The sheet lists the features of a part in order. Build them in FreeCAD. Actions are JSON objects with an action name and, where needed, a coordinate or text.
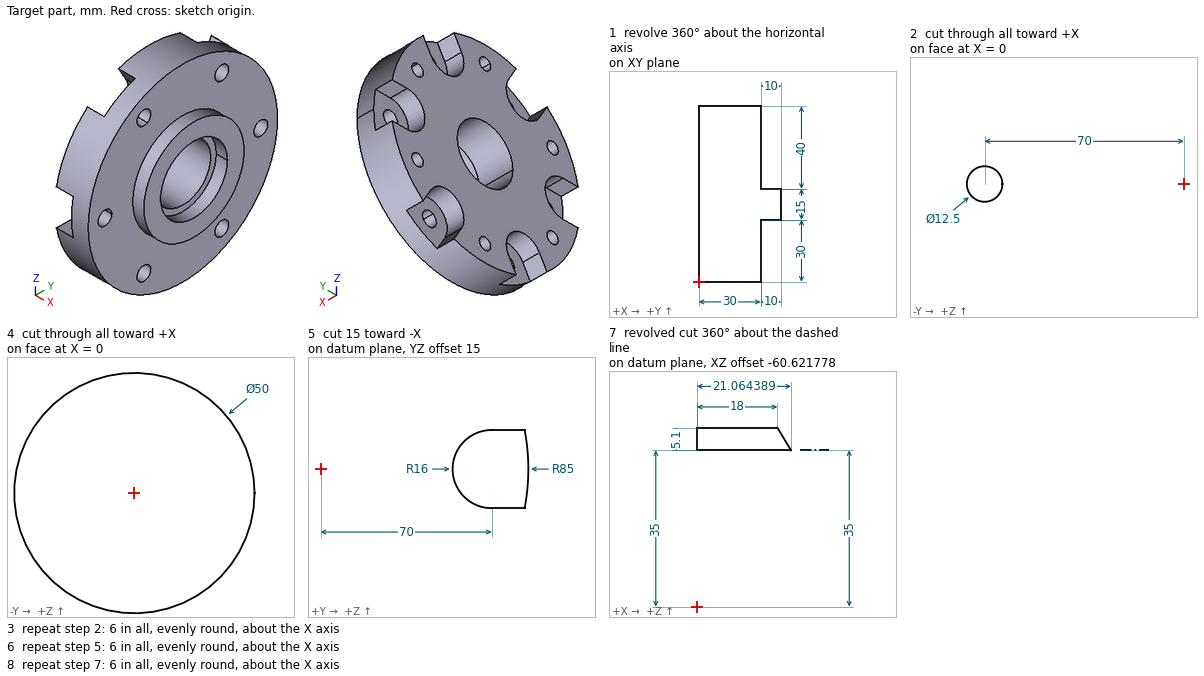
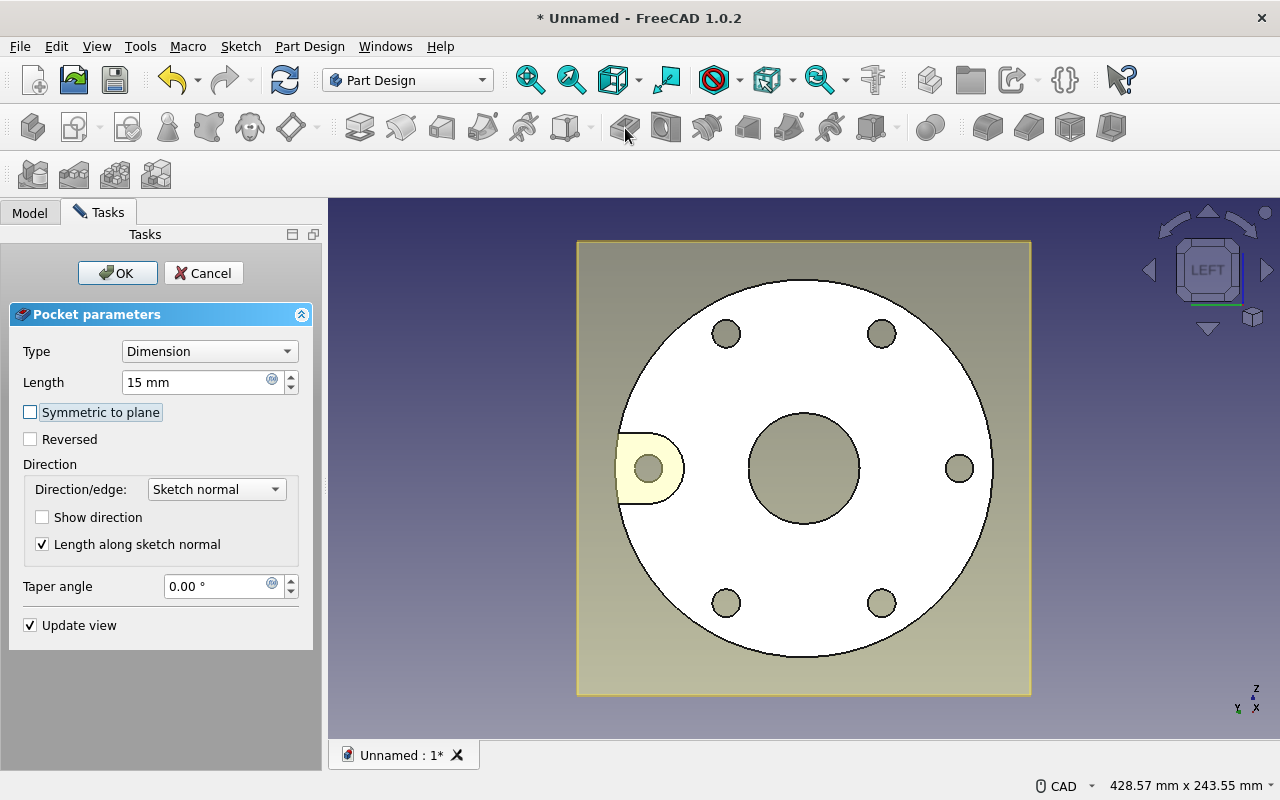
{"action": "left_click", "coordinate": [118, 273]}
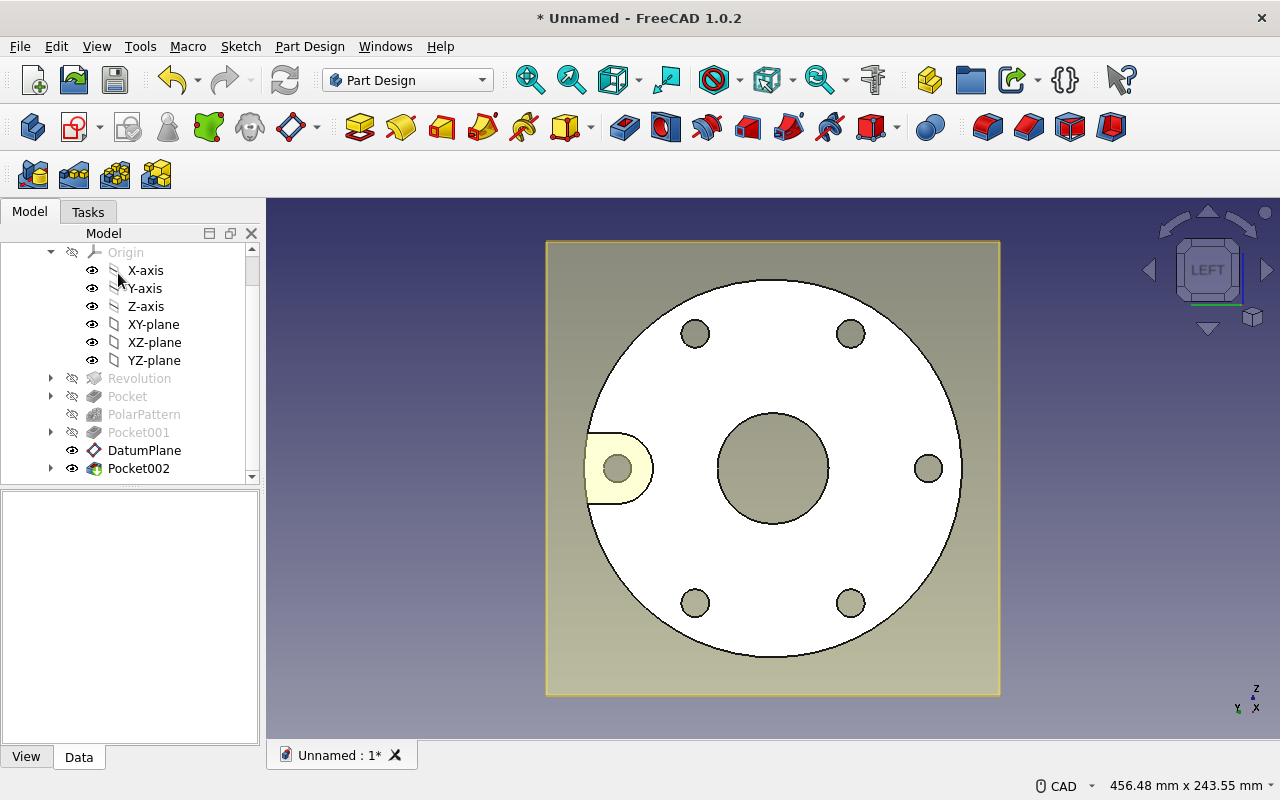
{"action": "left_click", "coordinate": [117, 450]}
{"action": "key", "text": "space"}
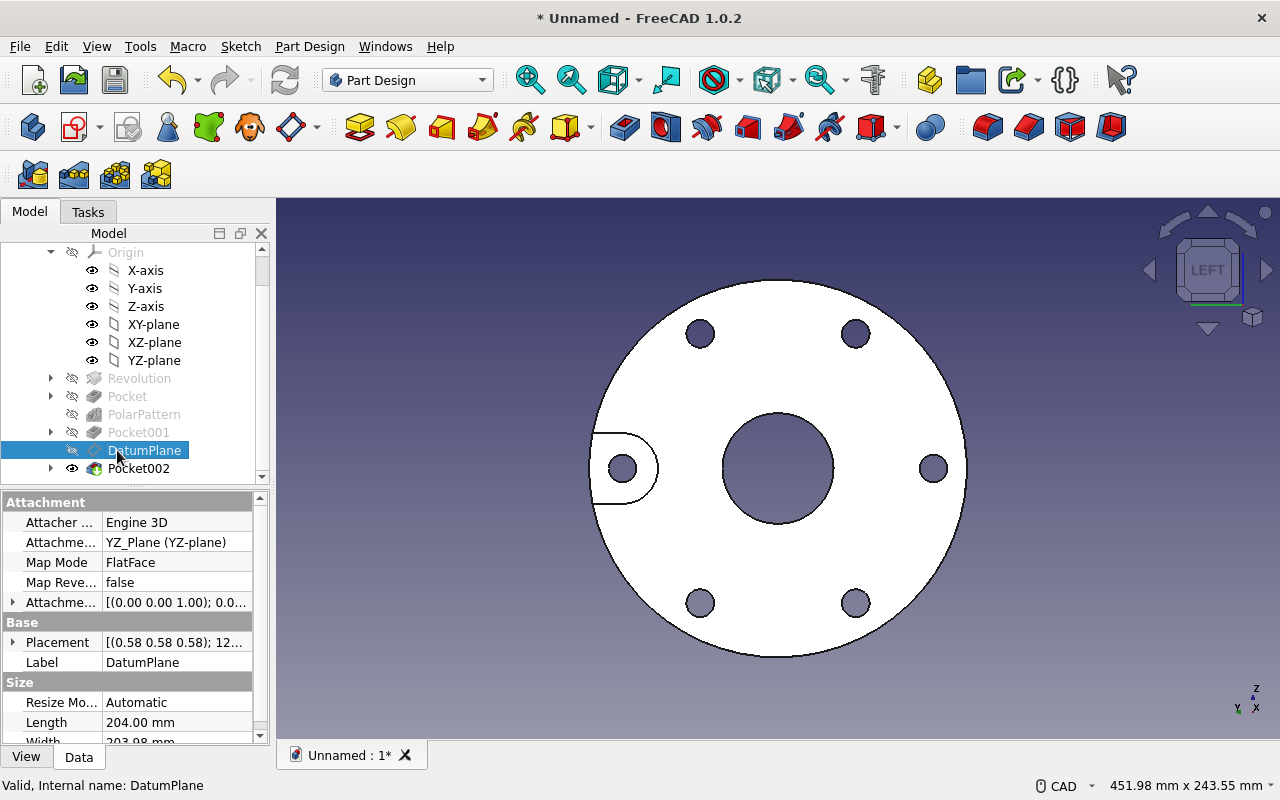
{"action": "left_click", "coordinate": [117, 468]}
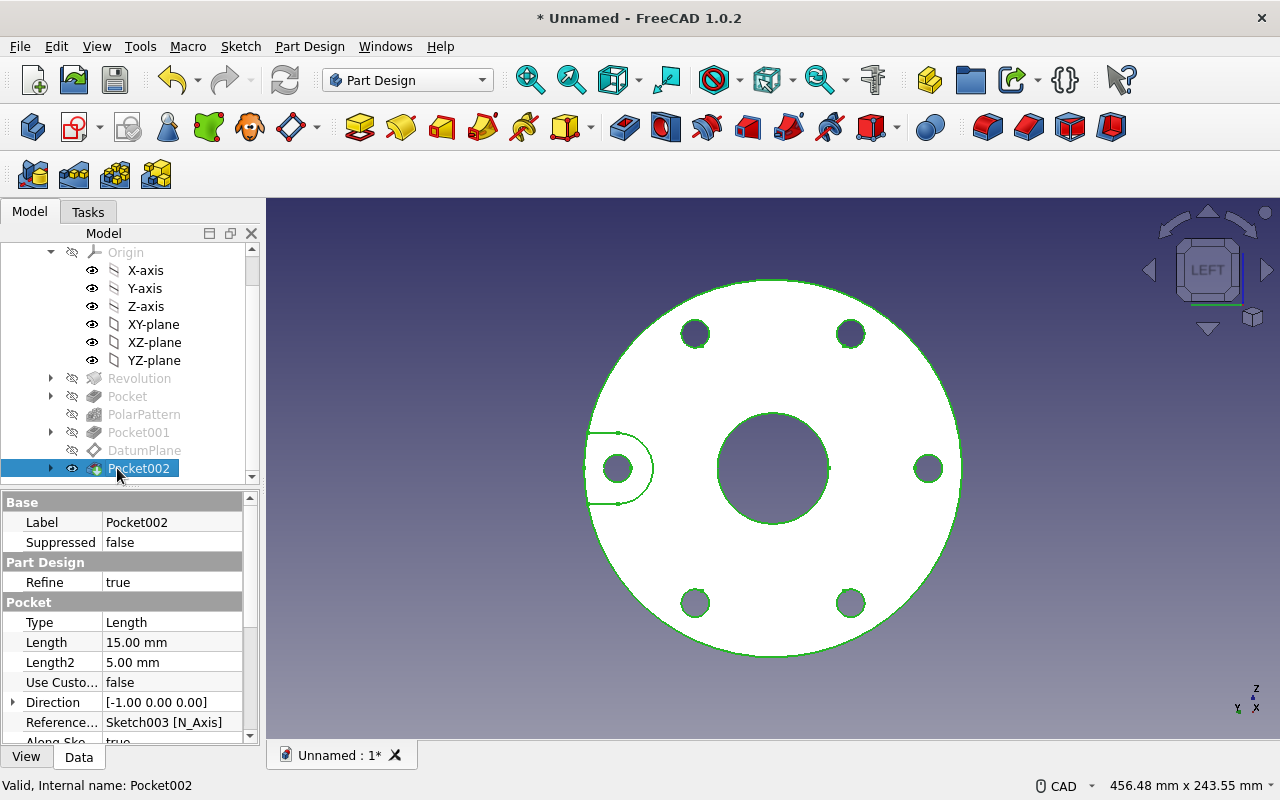
{"action": "left_click", "coordinate": [115, 174]}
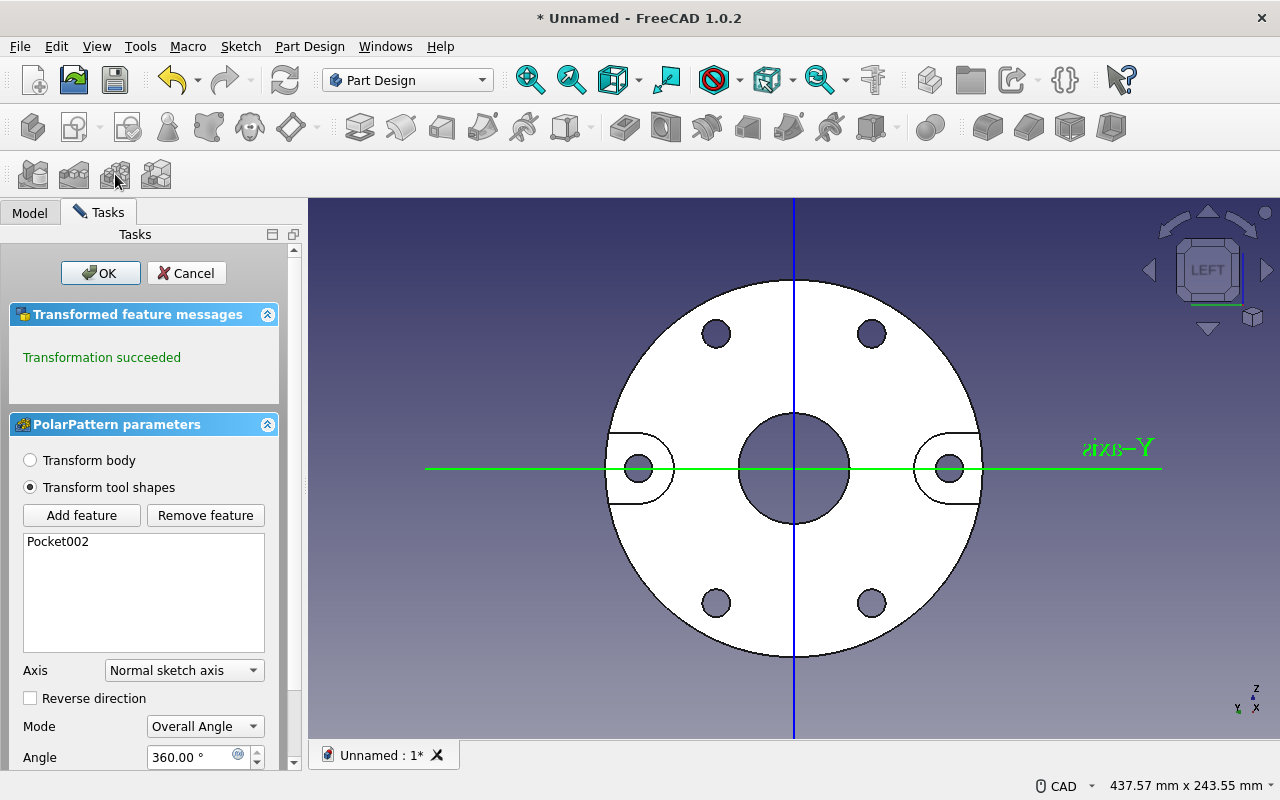
{"action": "left_click", "coordinate": [185, 670]}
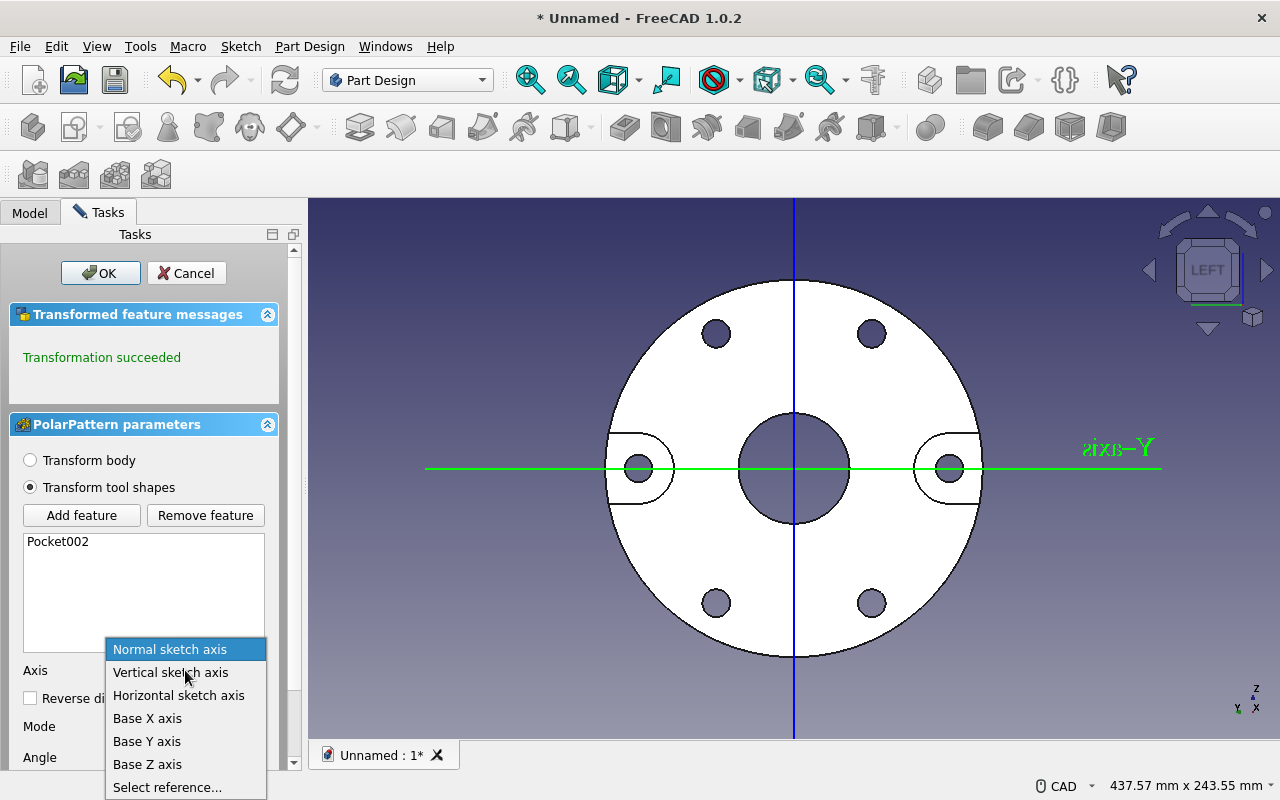
{"action": "left_click", "coordinate": [184, 718]}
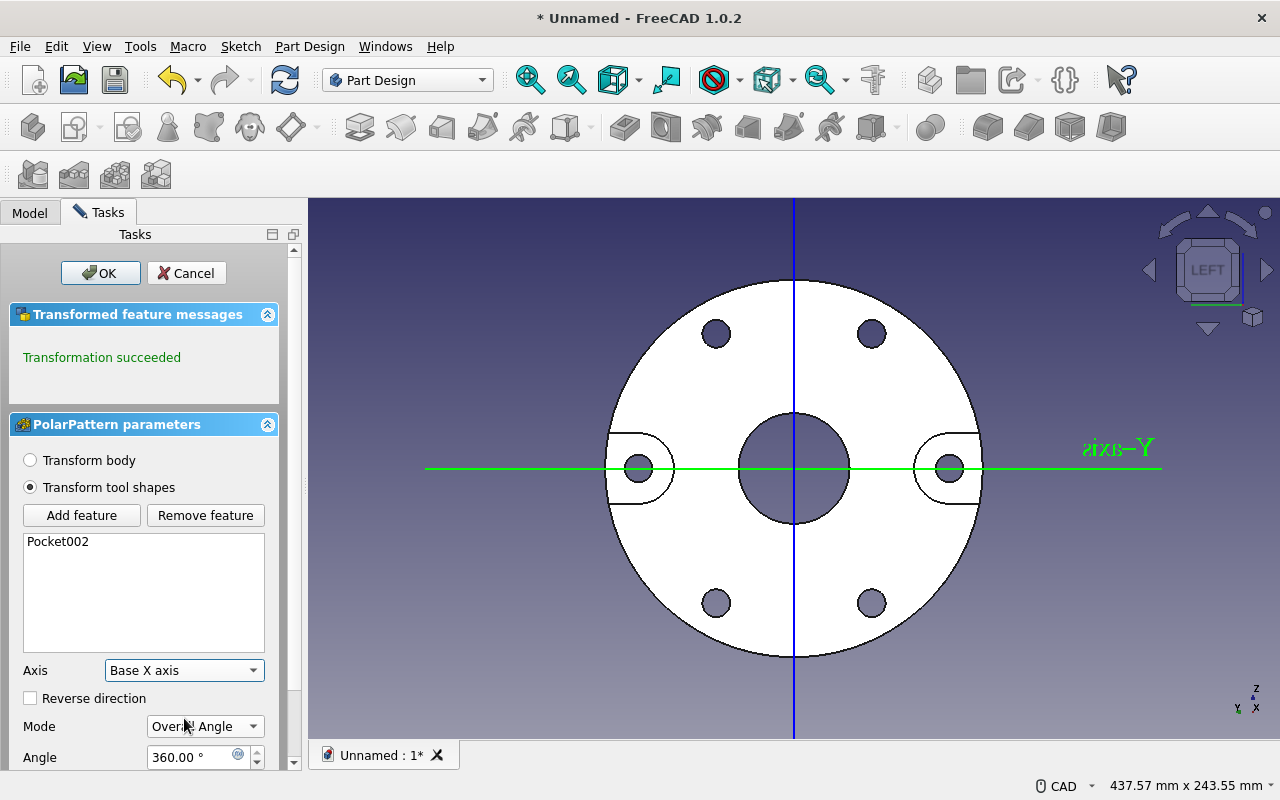
{"action": "scroll", "coordinate": [294, 507], "scroll_direction": "down", "scroll_amount": 2}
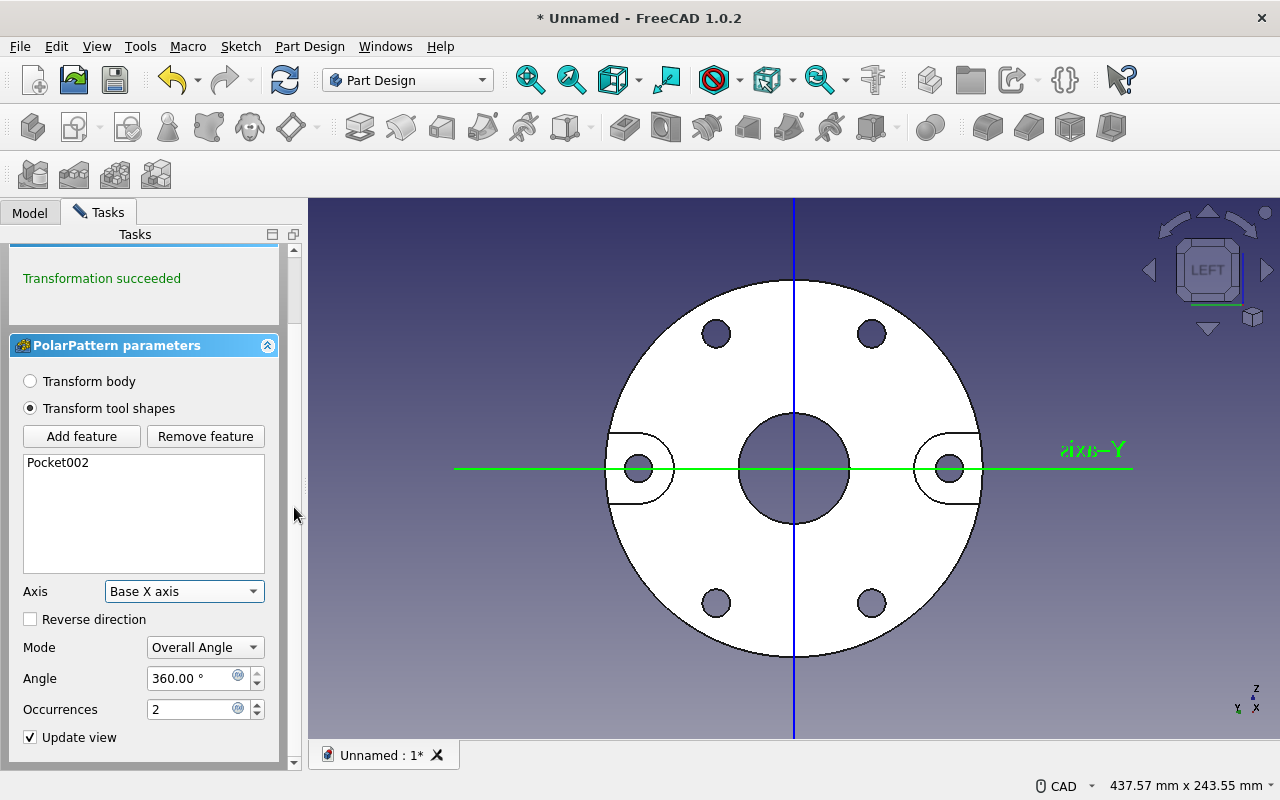
{"action": "triple_click", "coordinate": [199, 710]}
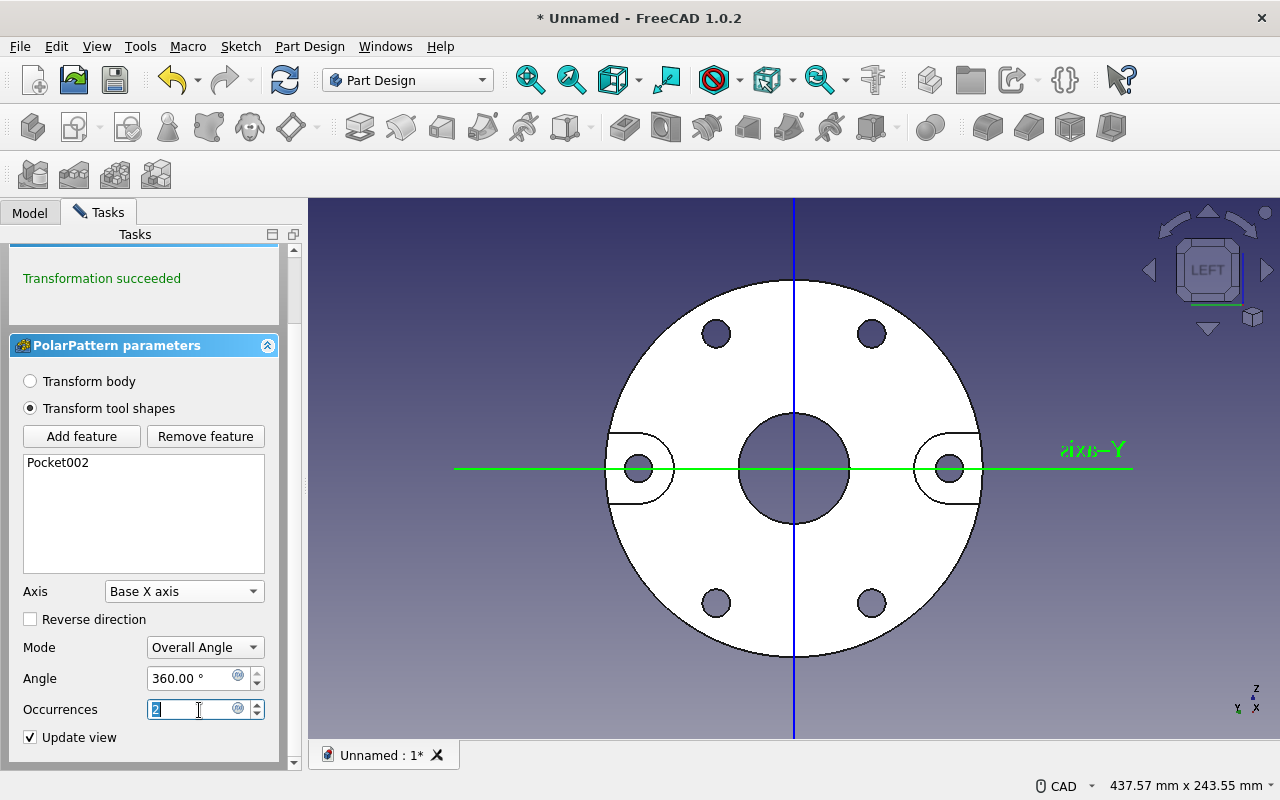
{"action": "type", "text": "6"}
{"action": "key", "text": "Tab"}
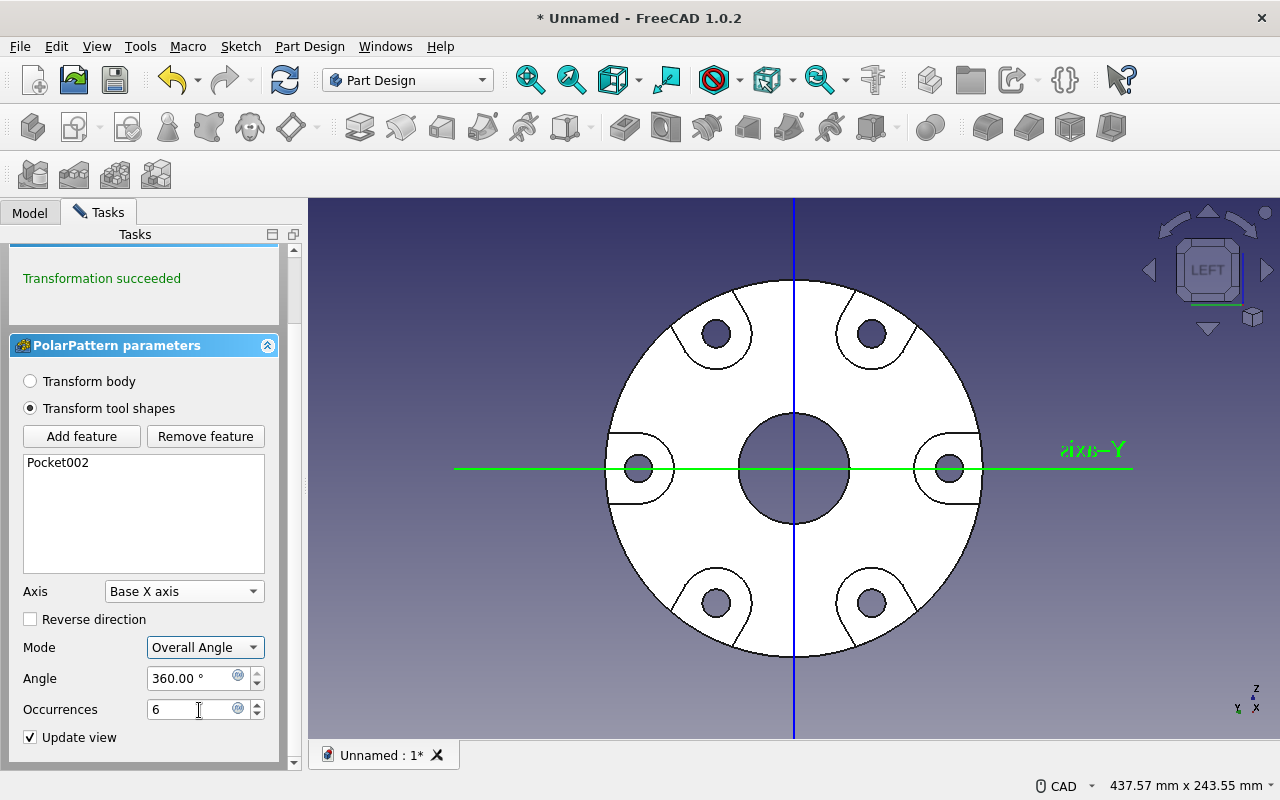
{"action": "scroll", "coordinate": [294, 507], "scroll_direction": "up", "scroll_amount": 3}